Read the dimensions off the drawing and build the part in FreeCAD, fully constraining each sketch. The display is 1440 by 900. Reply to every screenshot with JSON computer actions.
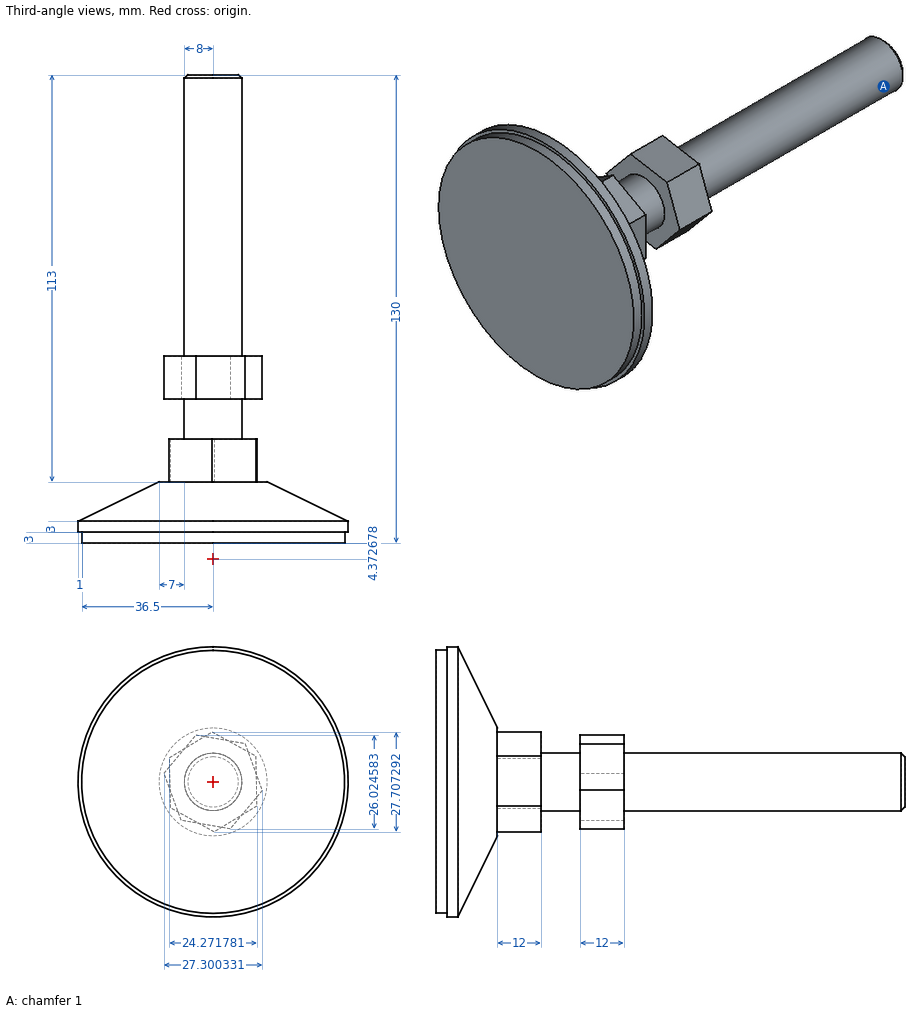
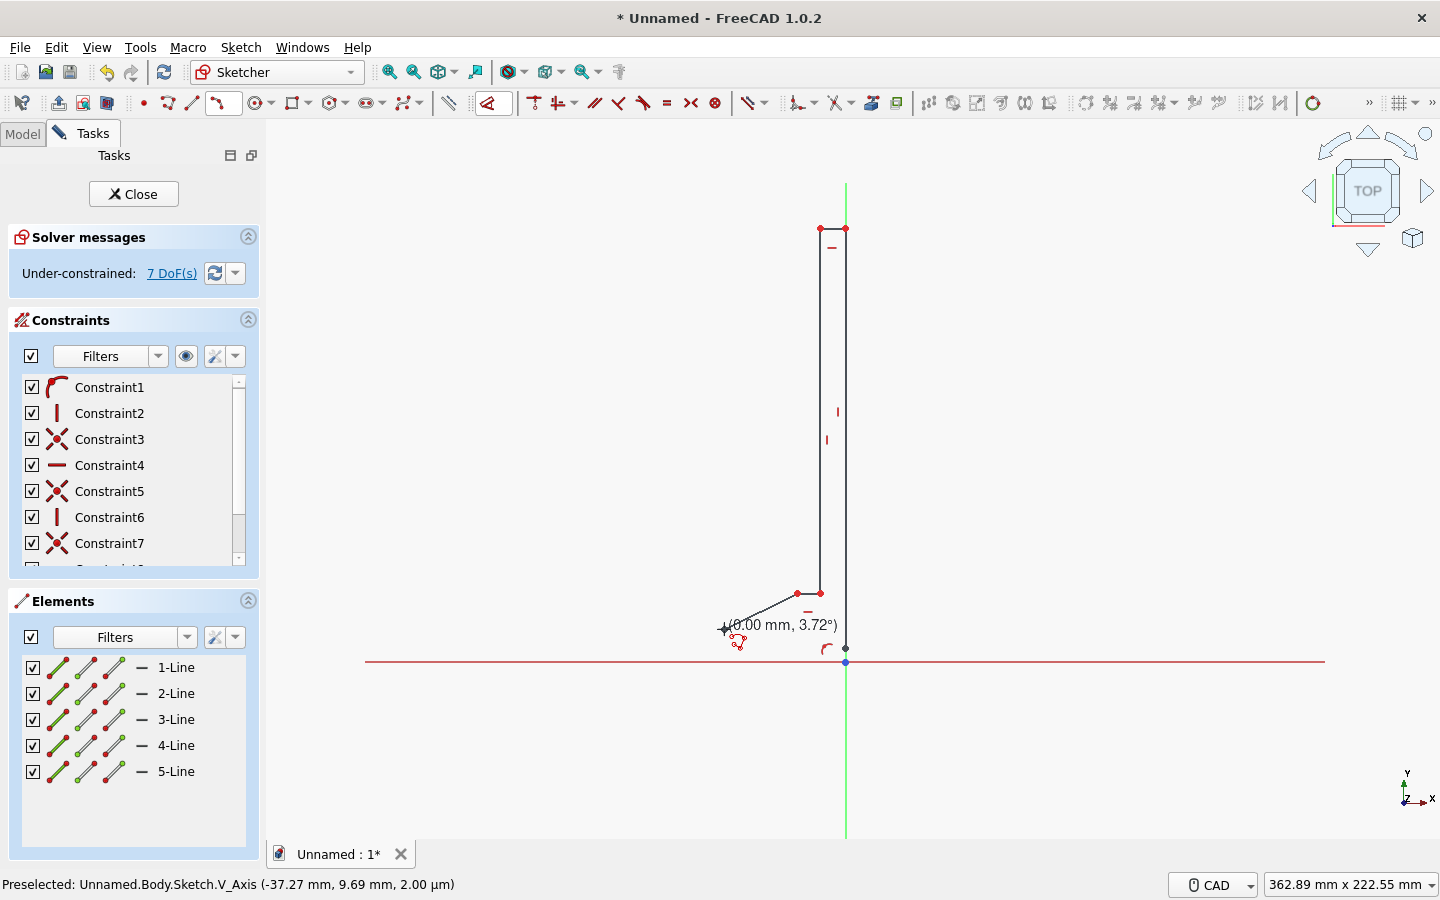
{"action": "scroll", "coordinate": [724, 639], "scroll_direction": "up", "scroll_amount": 3}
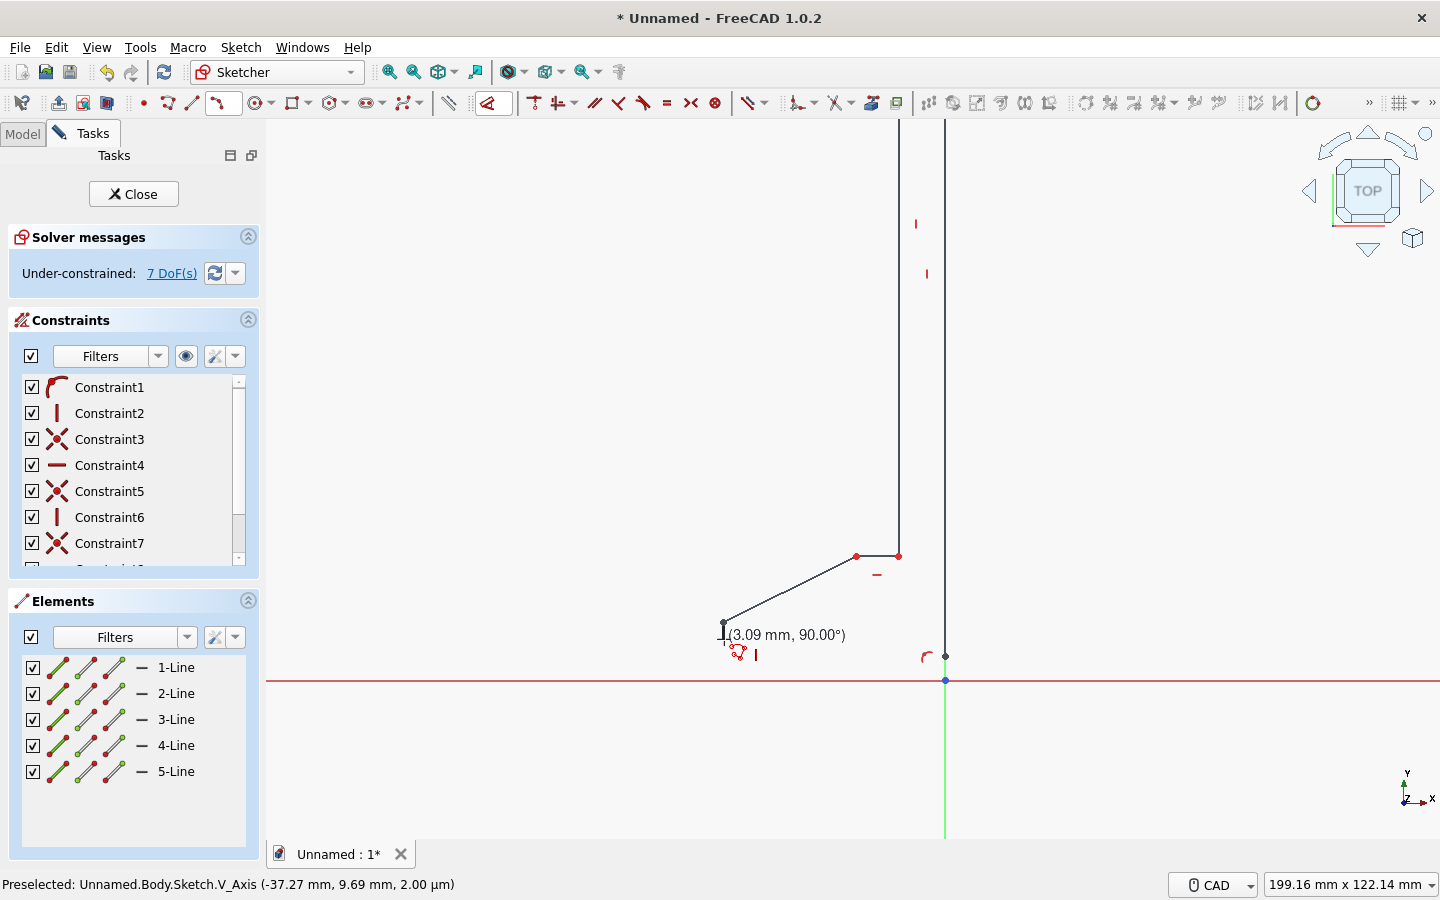
{"action": "left_click", "coordinate": [724, 637]}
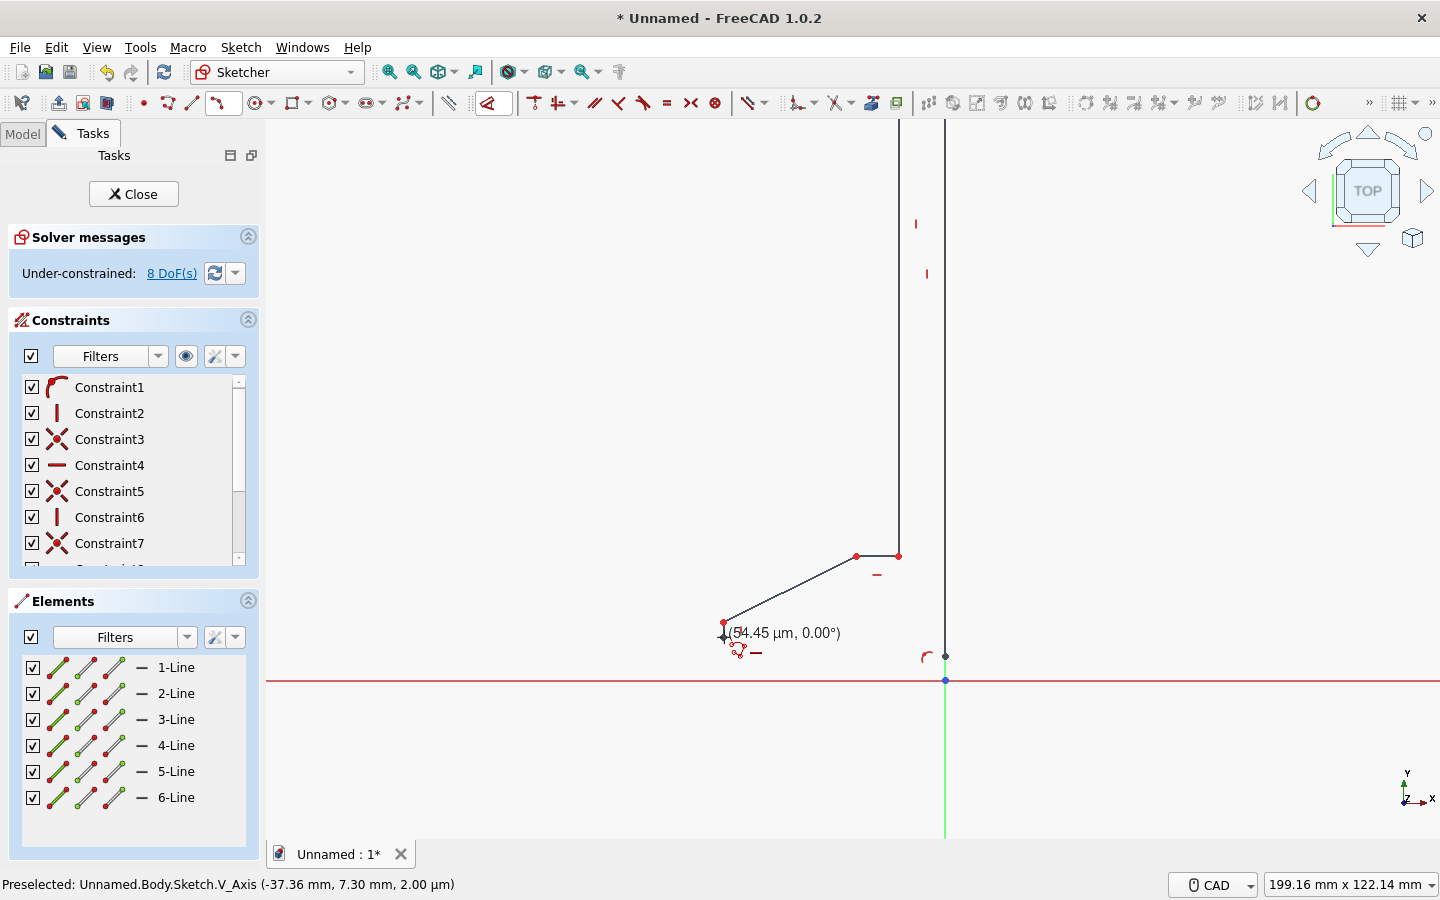
{"action": "scroll", "coordinate": [730, 637], "scroll_direction": "up", "scroll_amount": 5}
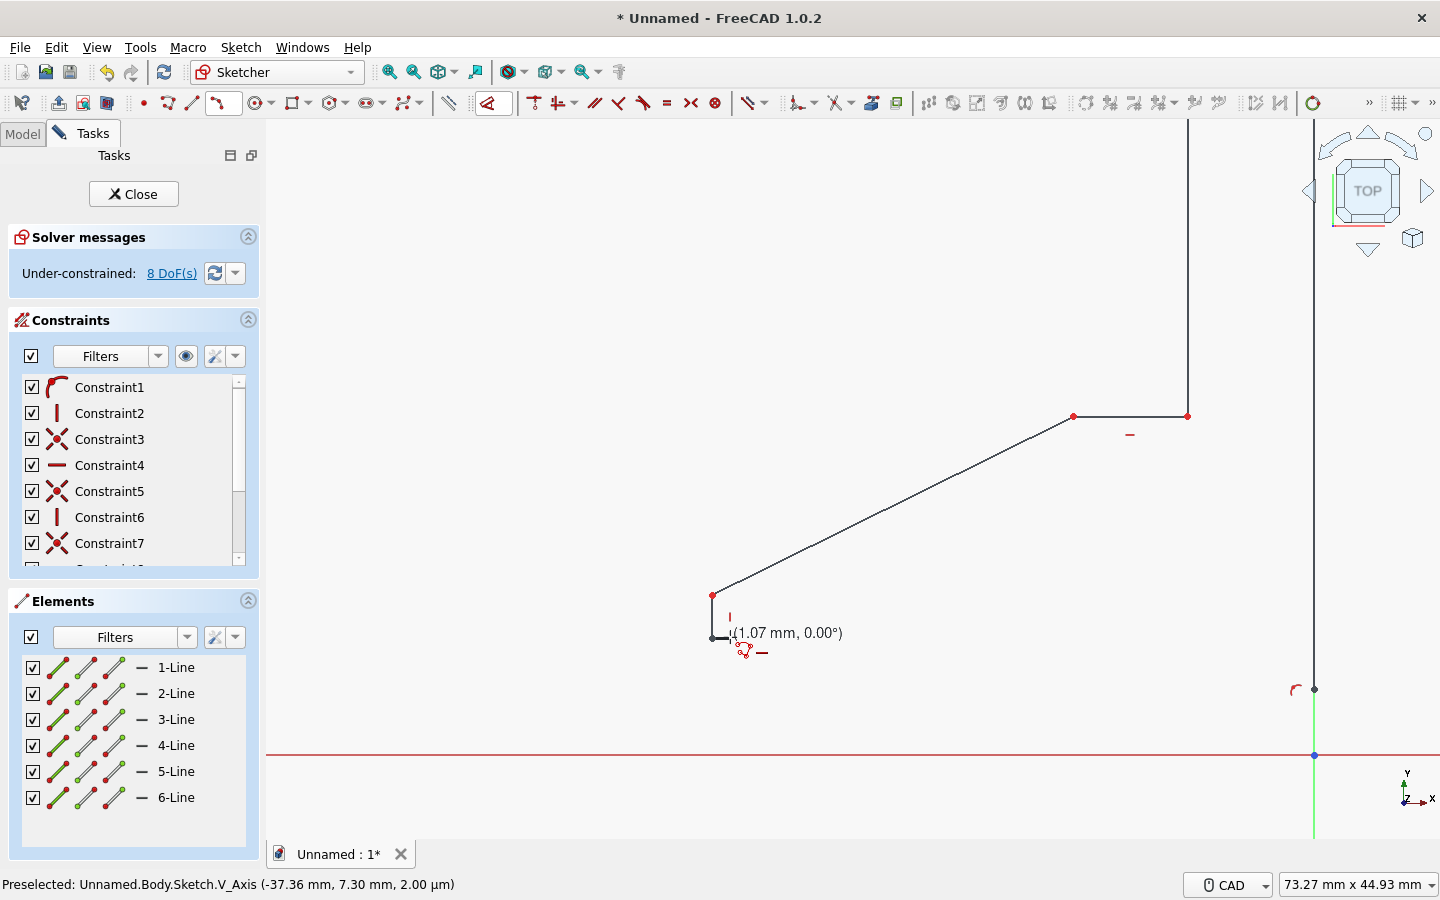
{"action": "left_click", "coordinate": [729, 636]}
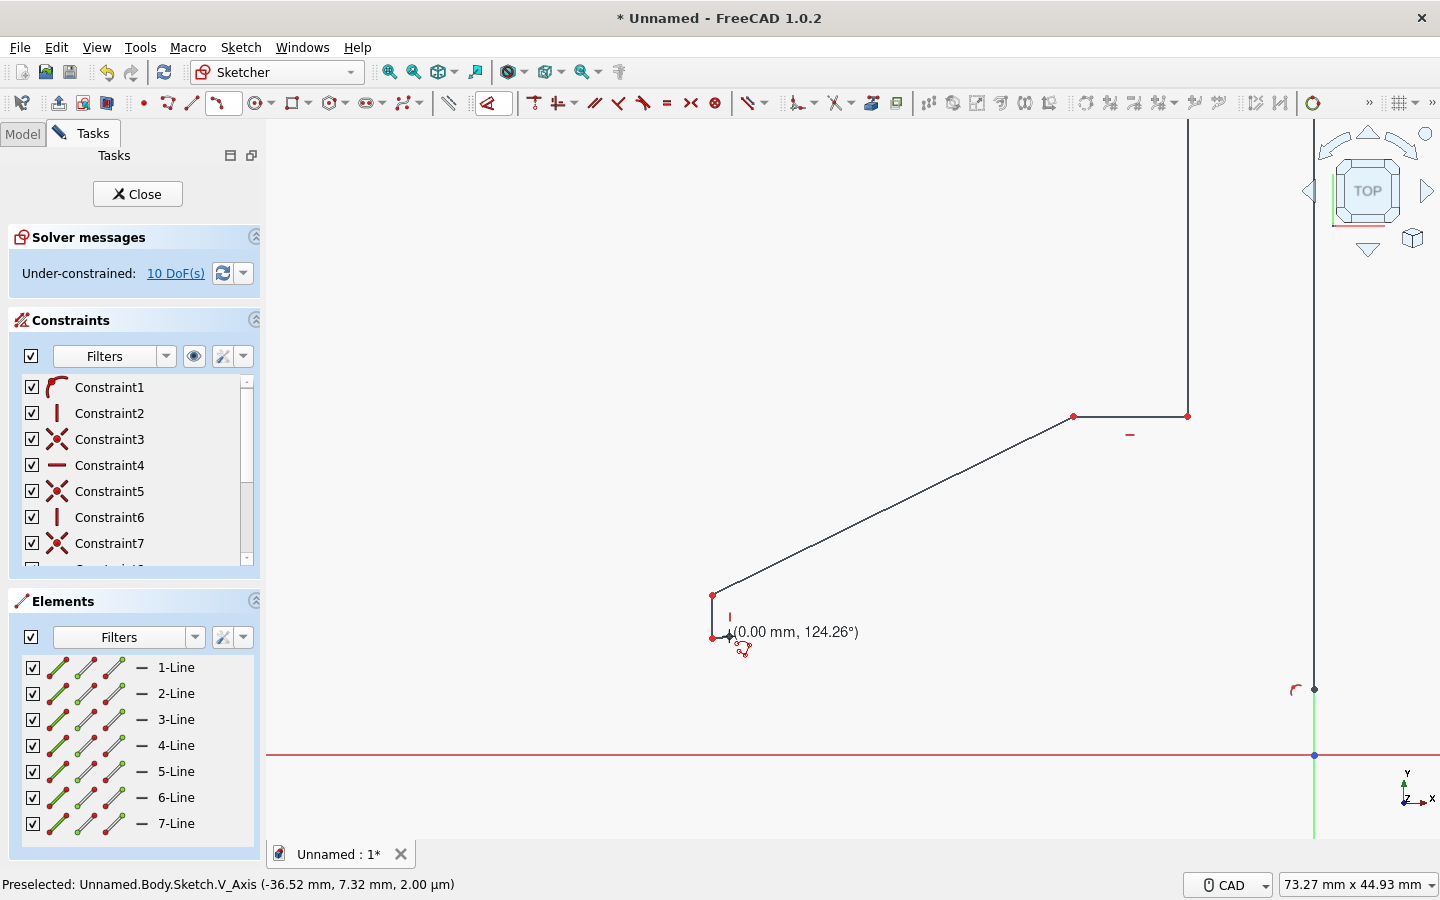
{"action": "scroll", "coordinate": [726, 681], "scroll_direction": "down", "scroll_amount": 8}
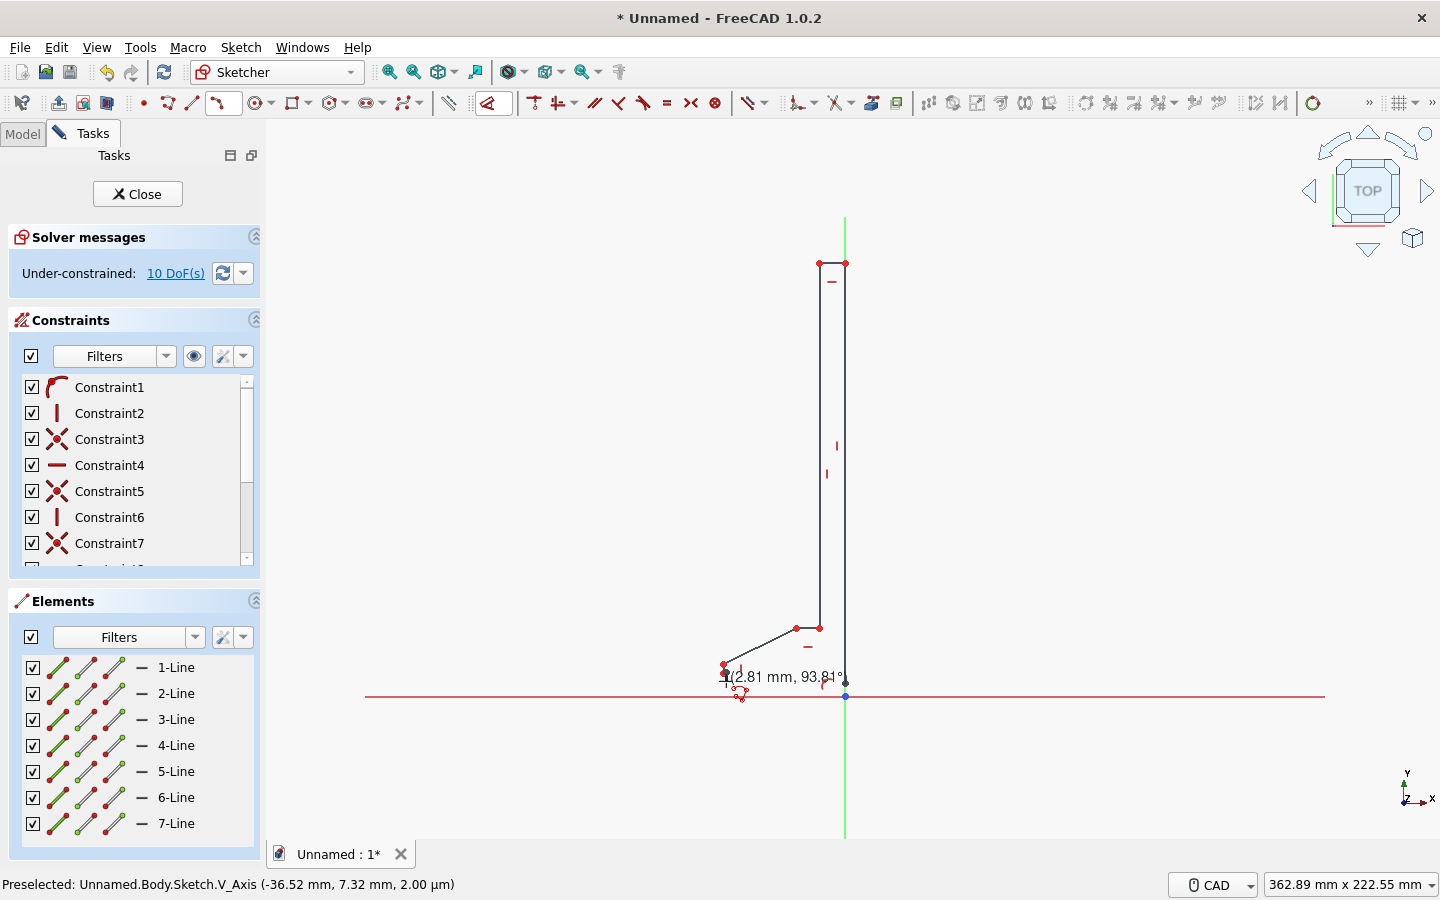
{"action": "scroll", "coordinate": [727, 682], "scroll_direction": "up", "scroll_amount": 3}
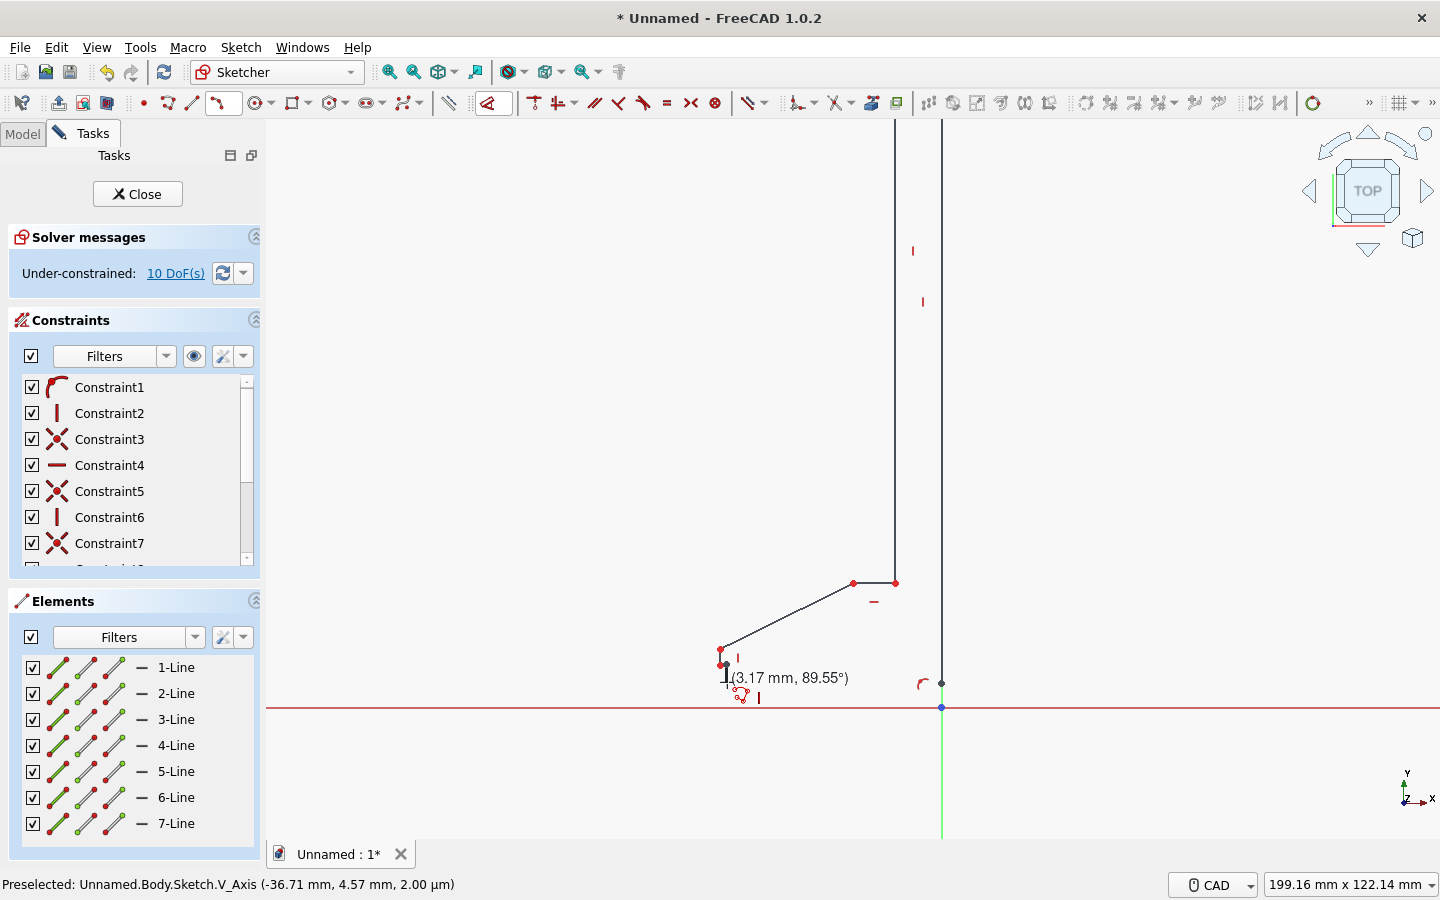
{"action": "left_click", "coordinate": [727, 682]}
{"action": "left_click", "coordinate": [942, 684]}
{"action": "key", "text": "Escape"}
{"action": "key", "text": "Escape"}